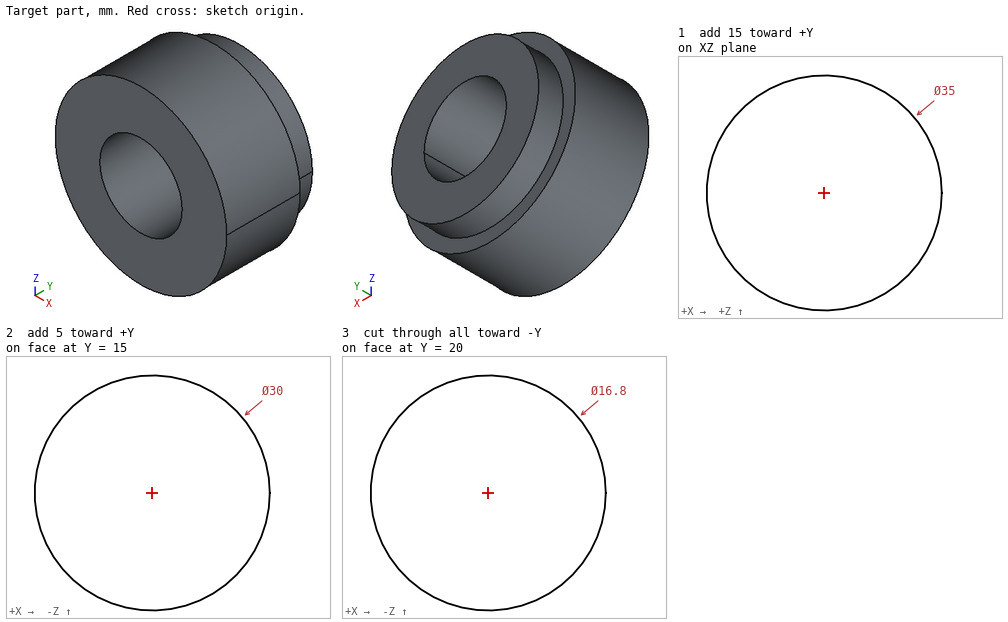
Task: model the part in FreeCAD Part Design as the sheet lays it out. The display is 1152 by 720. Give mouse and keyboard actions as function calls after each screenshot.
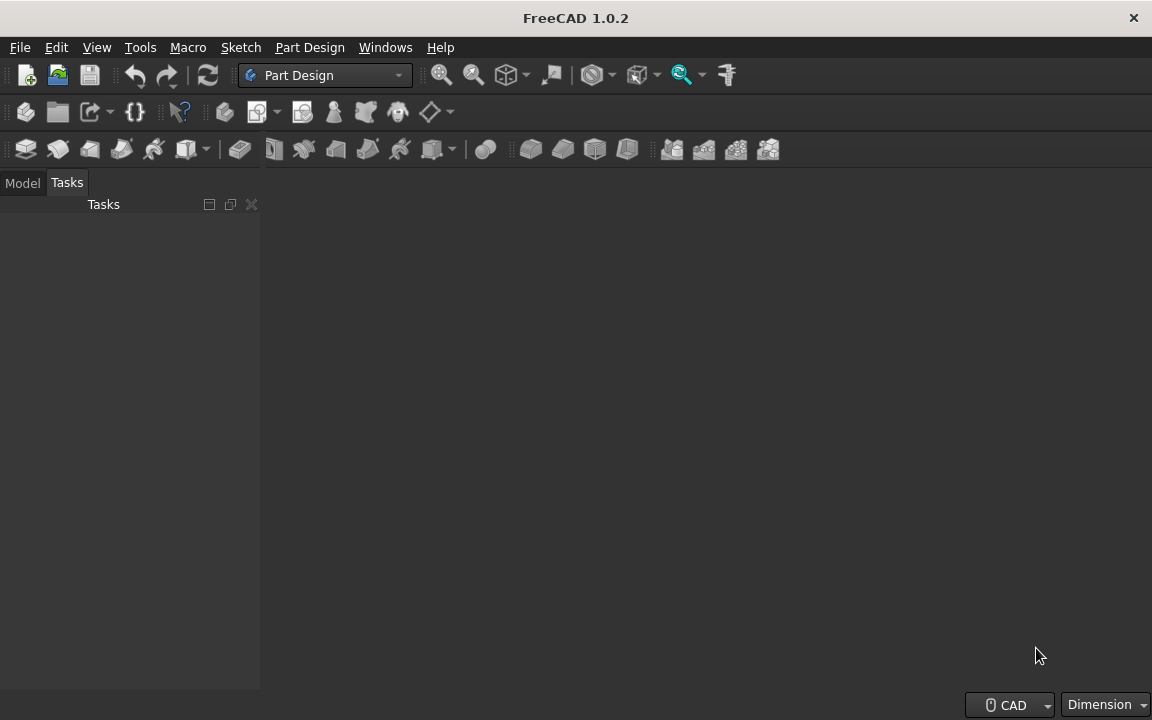
click(26, 76)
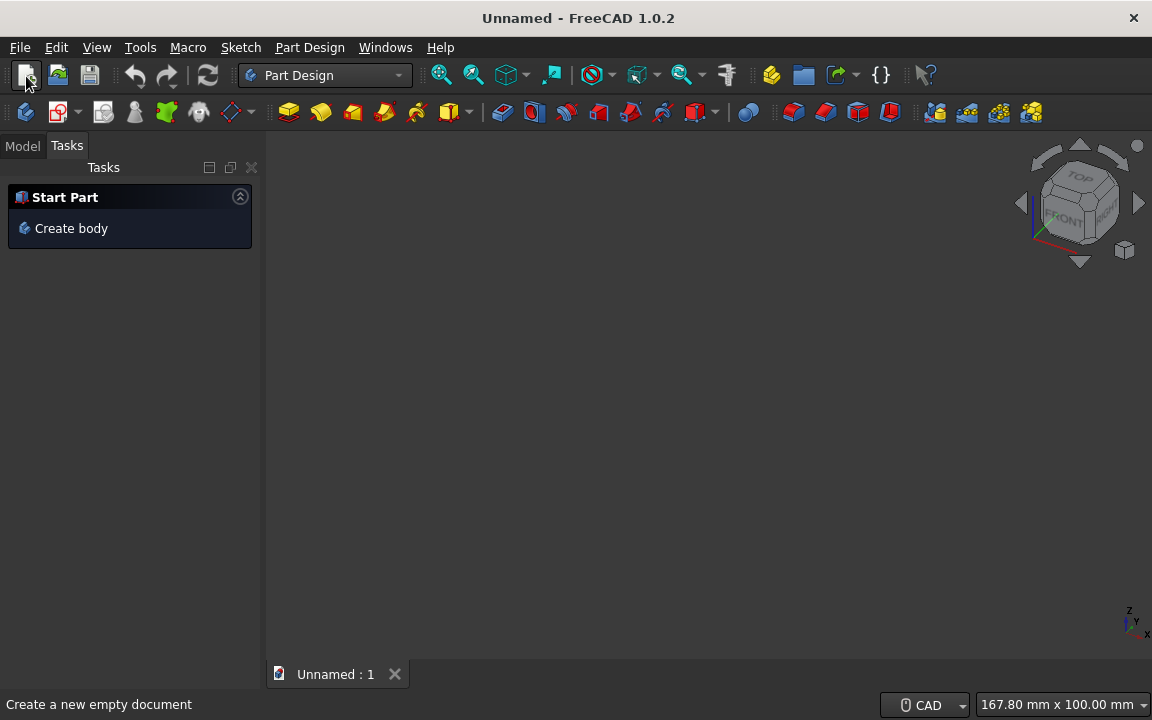
click(58, 112)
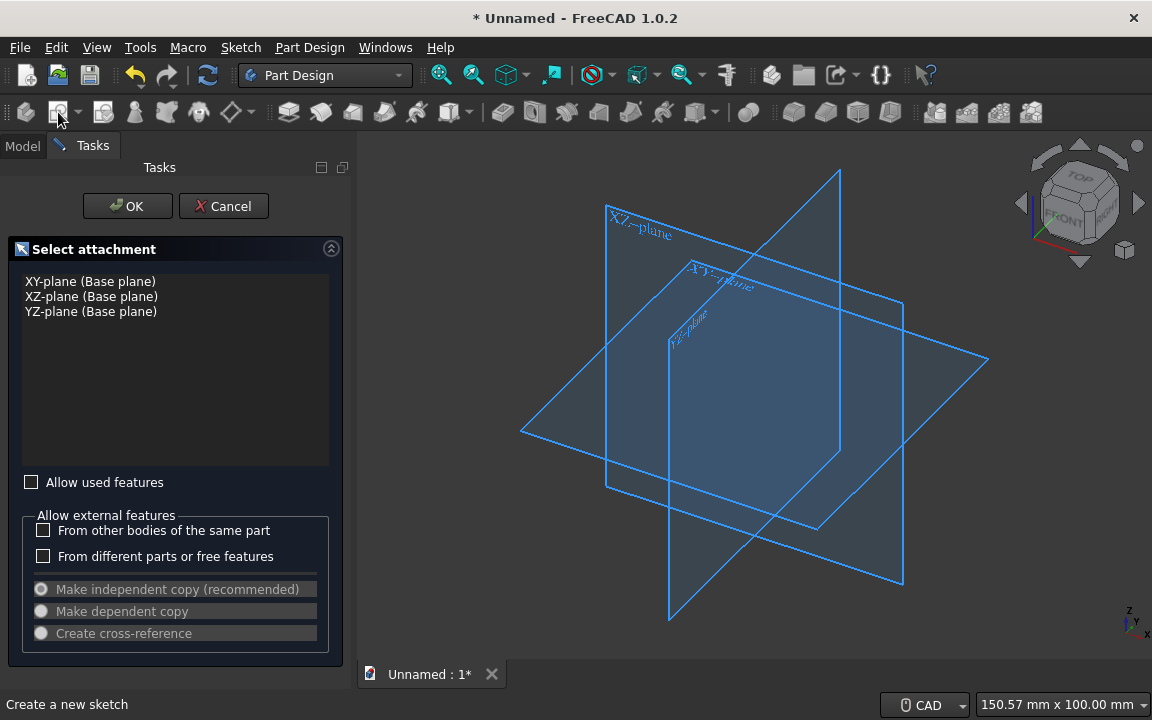
click(82, 296)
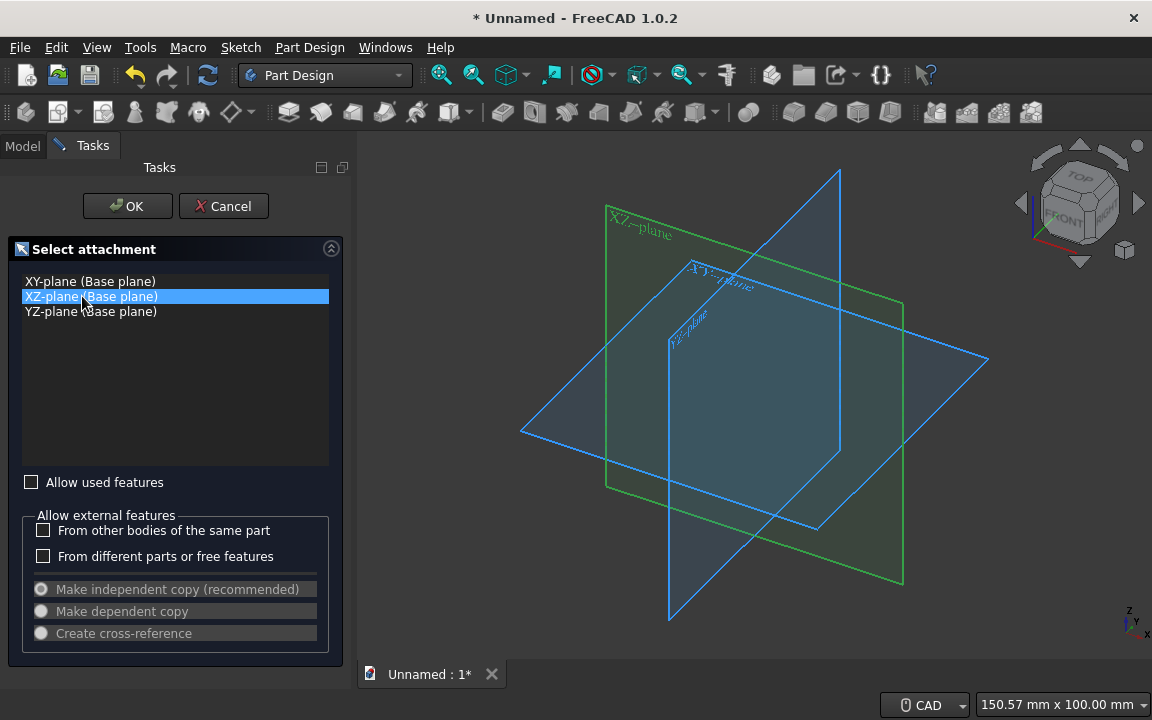
click(128, 206)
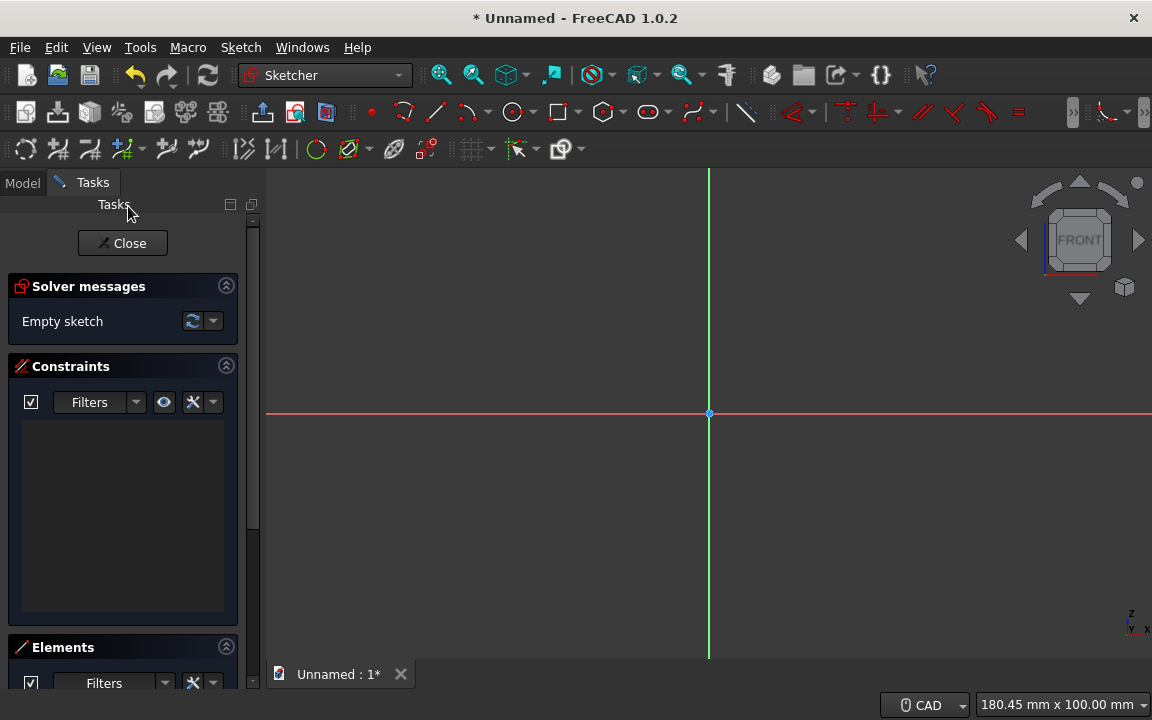
scroll(792, 414, up, 3)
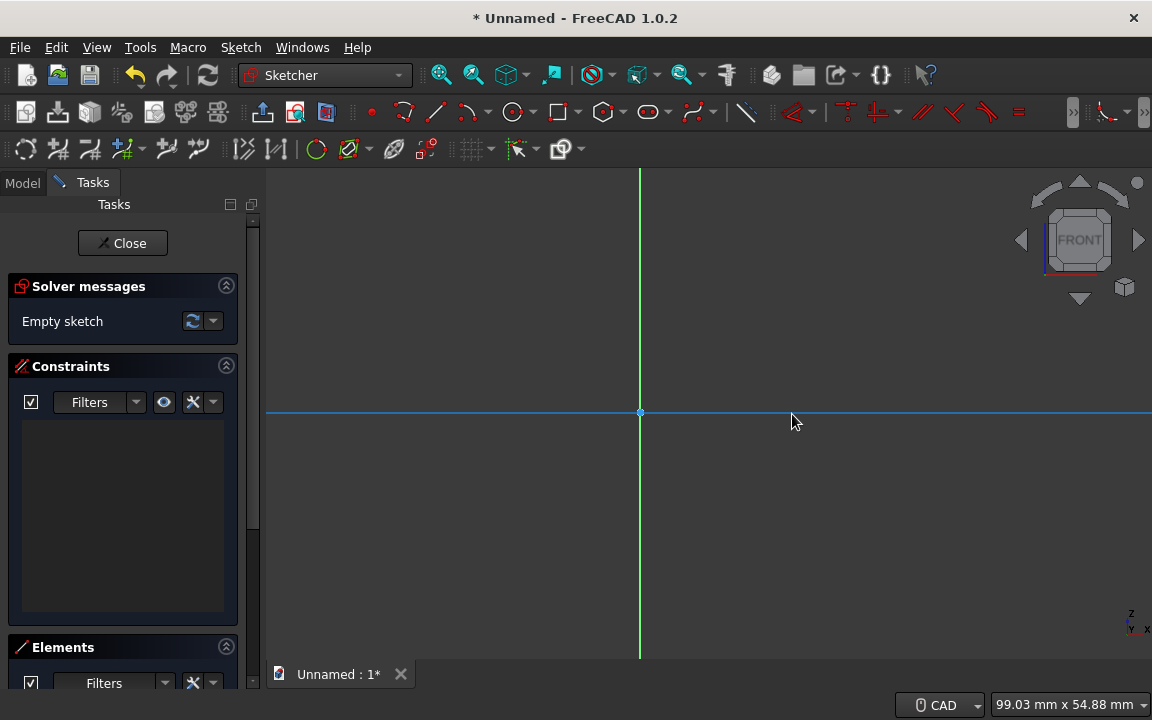
click(514, 112)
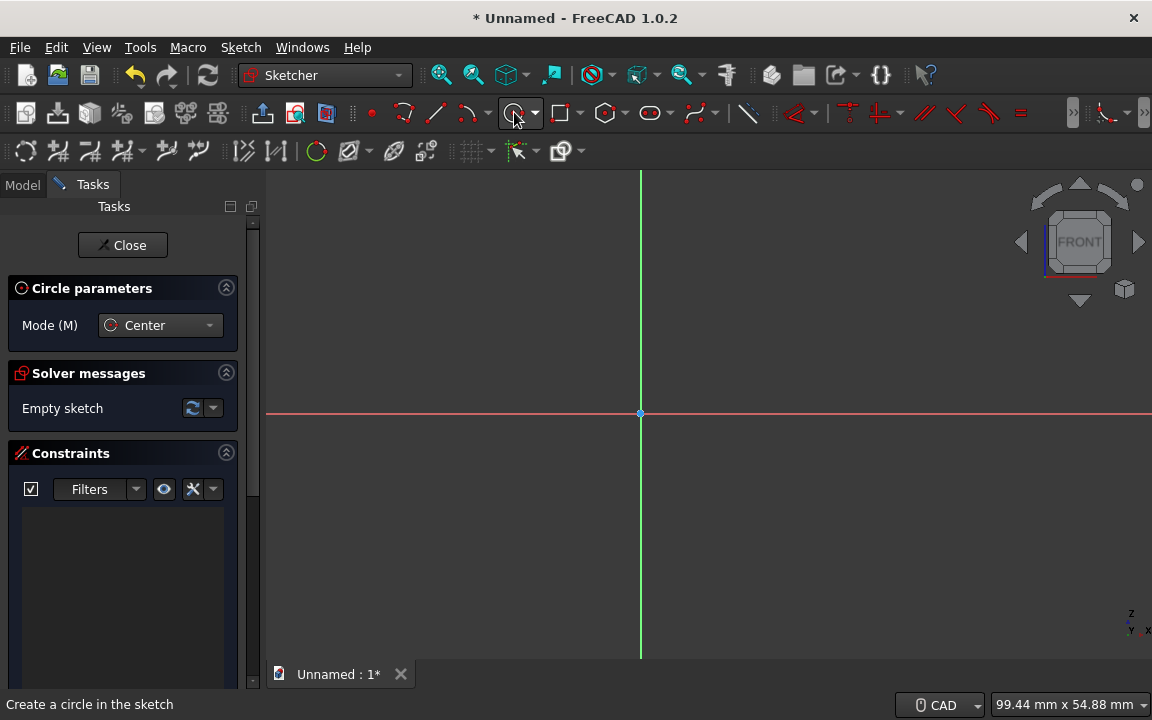
click(641, 414)
click(751, 303)
key(Escape)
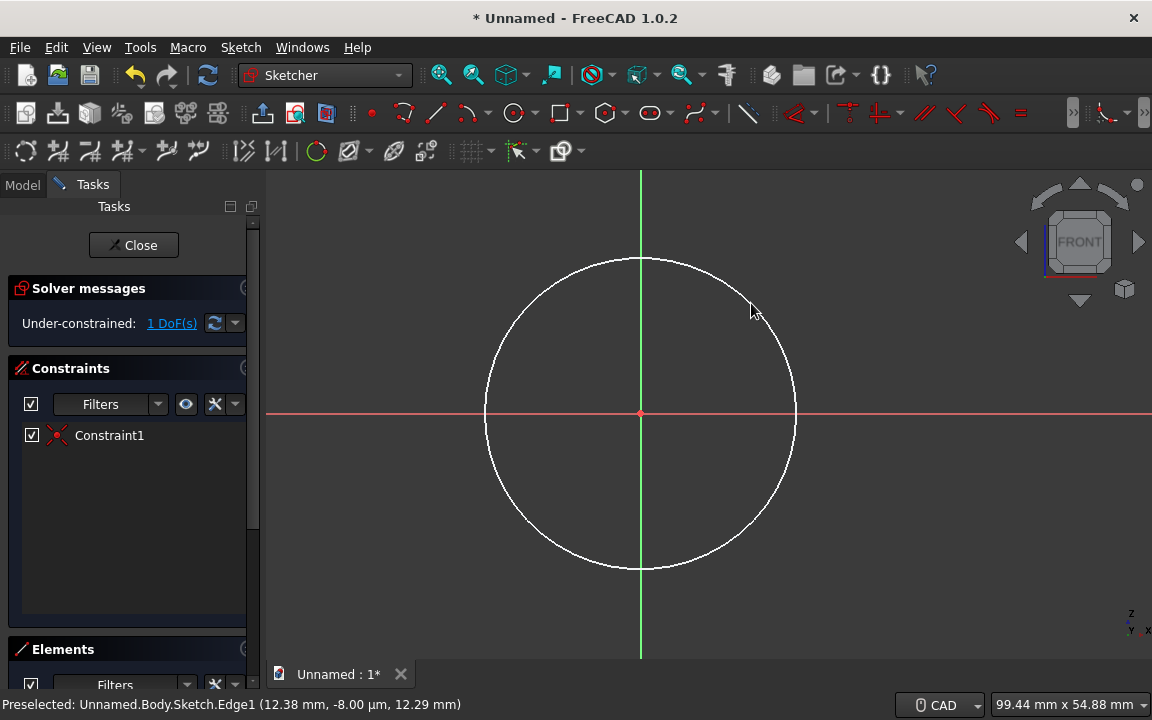
click(794, 114)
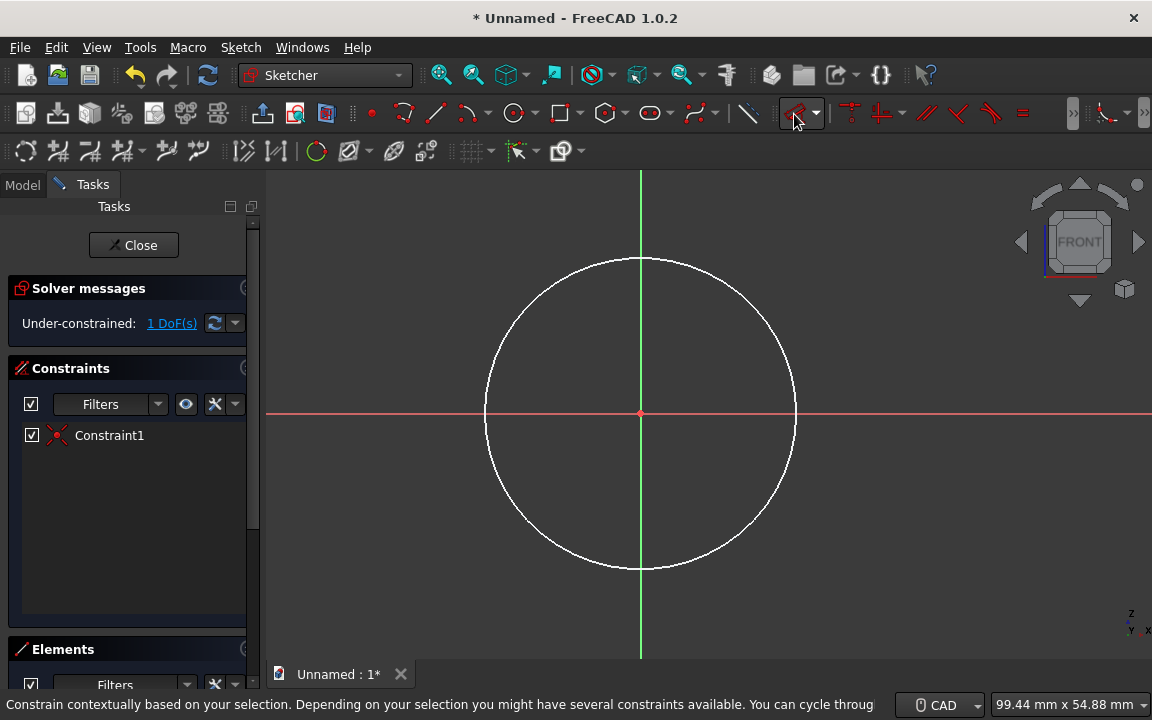
click(750, 303)
click(773, 280)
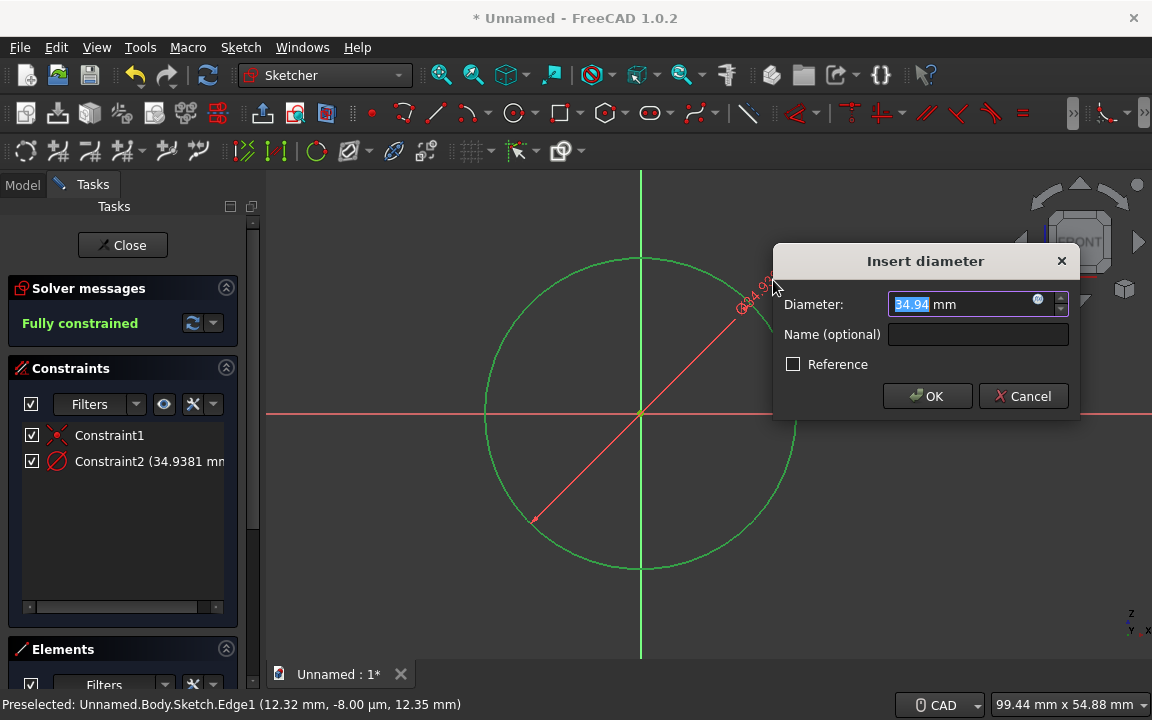
text(35)
key(Return)
key(Escape)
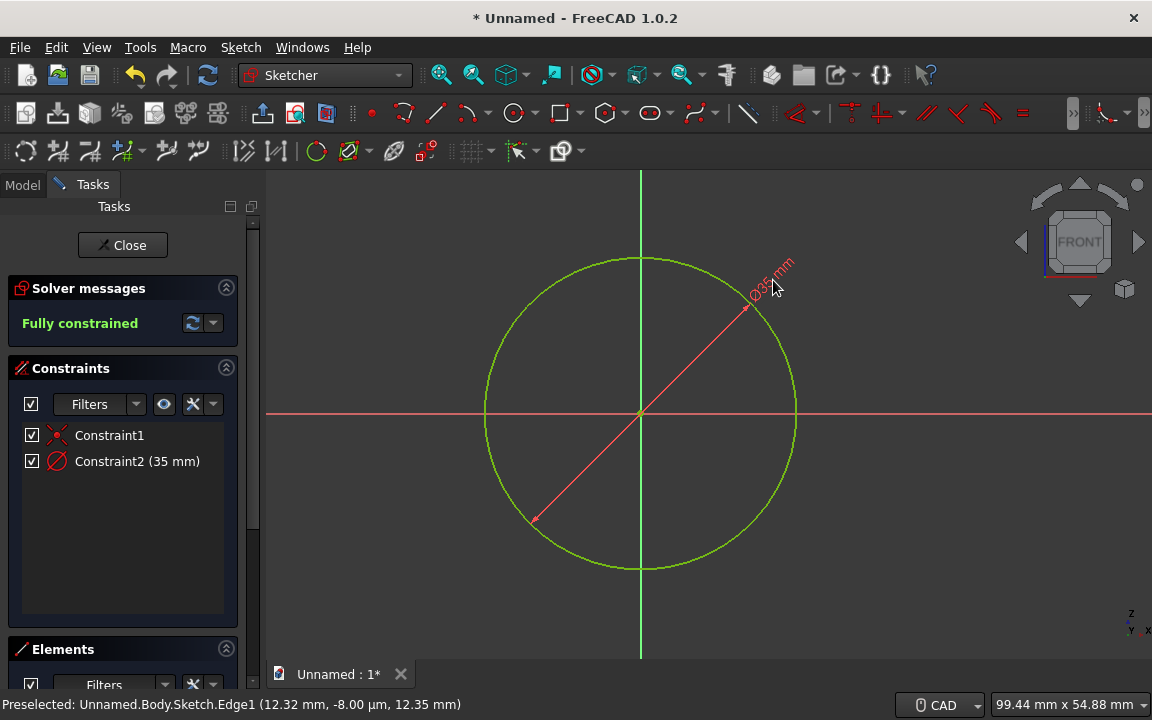
click(123, 245)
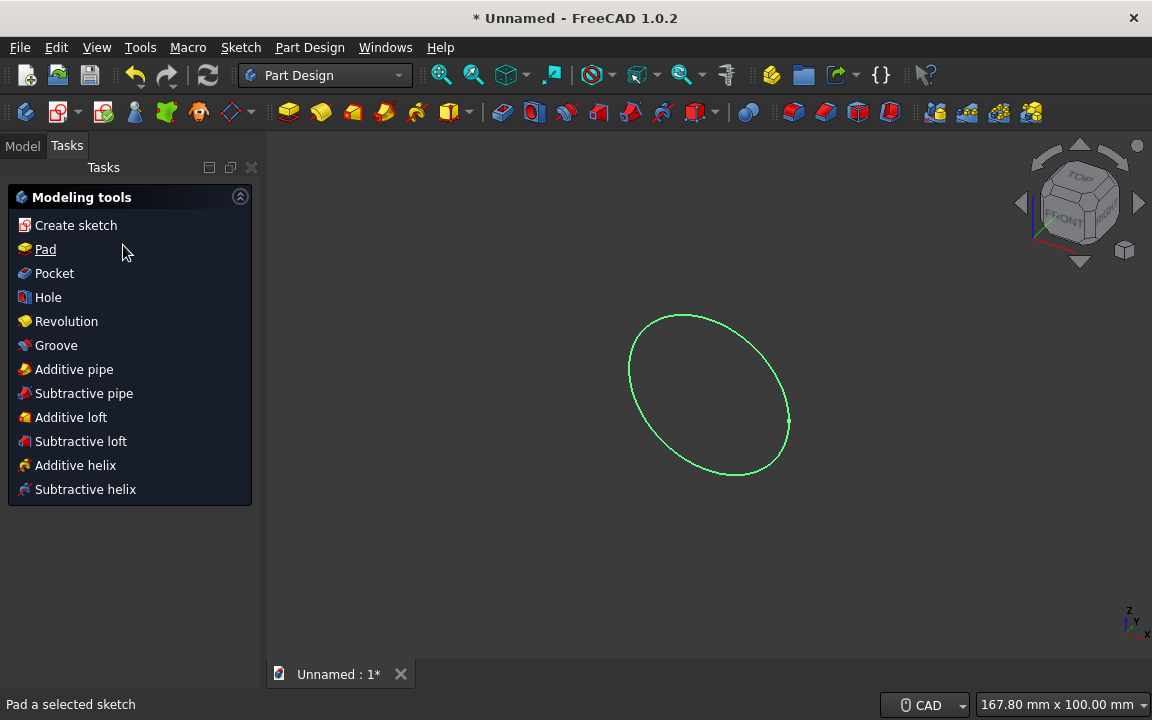
click(290, 112)